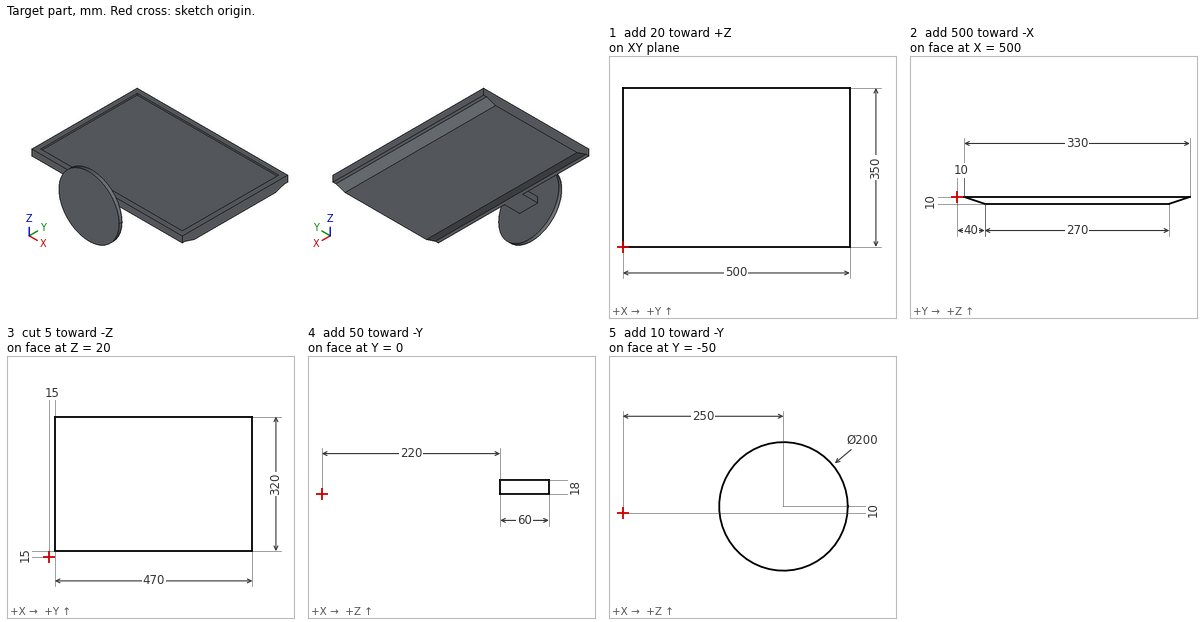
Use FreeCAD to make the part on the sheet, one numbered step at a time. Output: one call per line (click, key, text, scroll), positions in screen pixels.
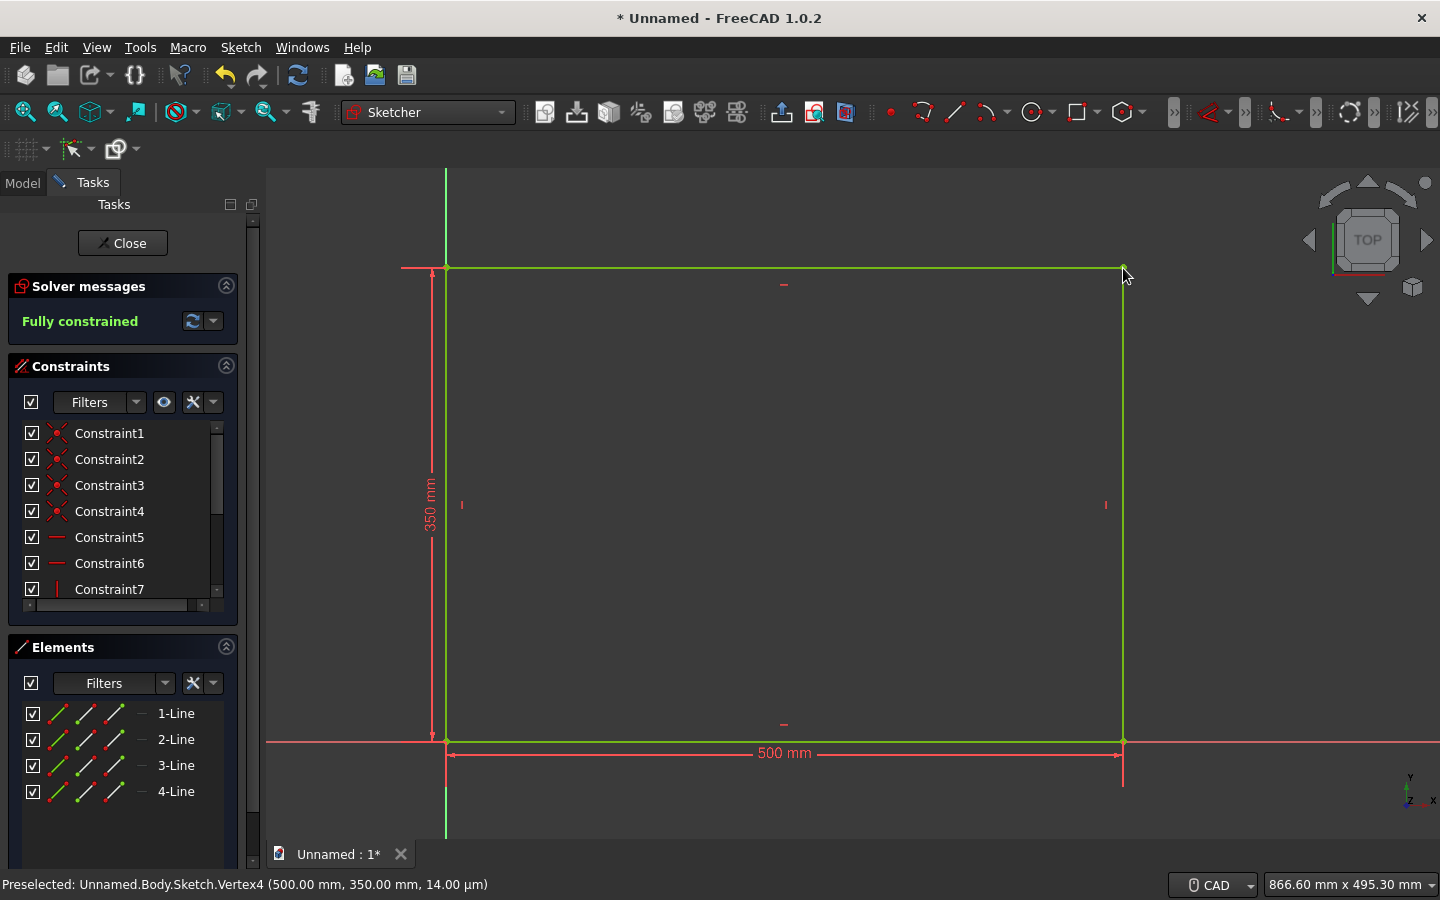
click(123, 243)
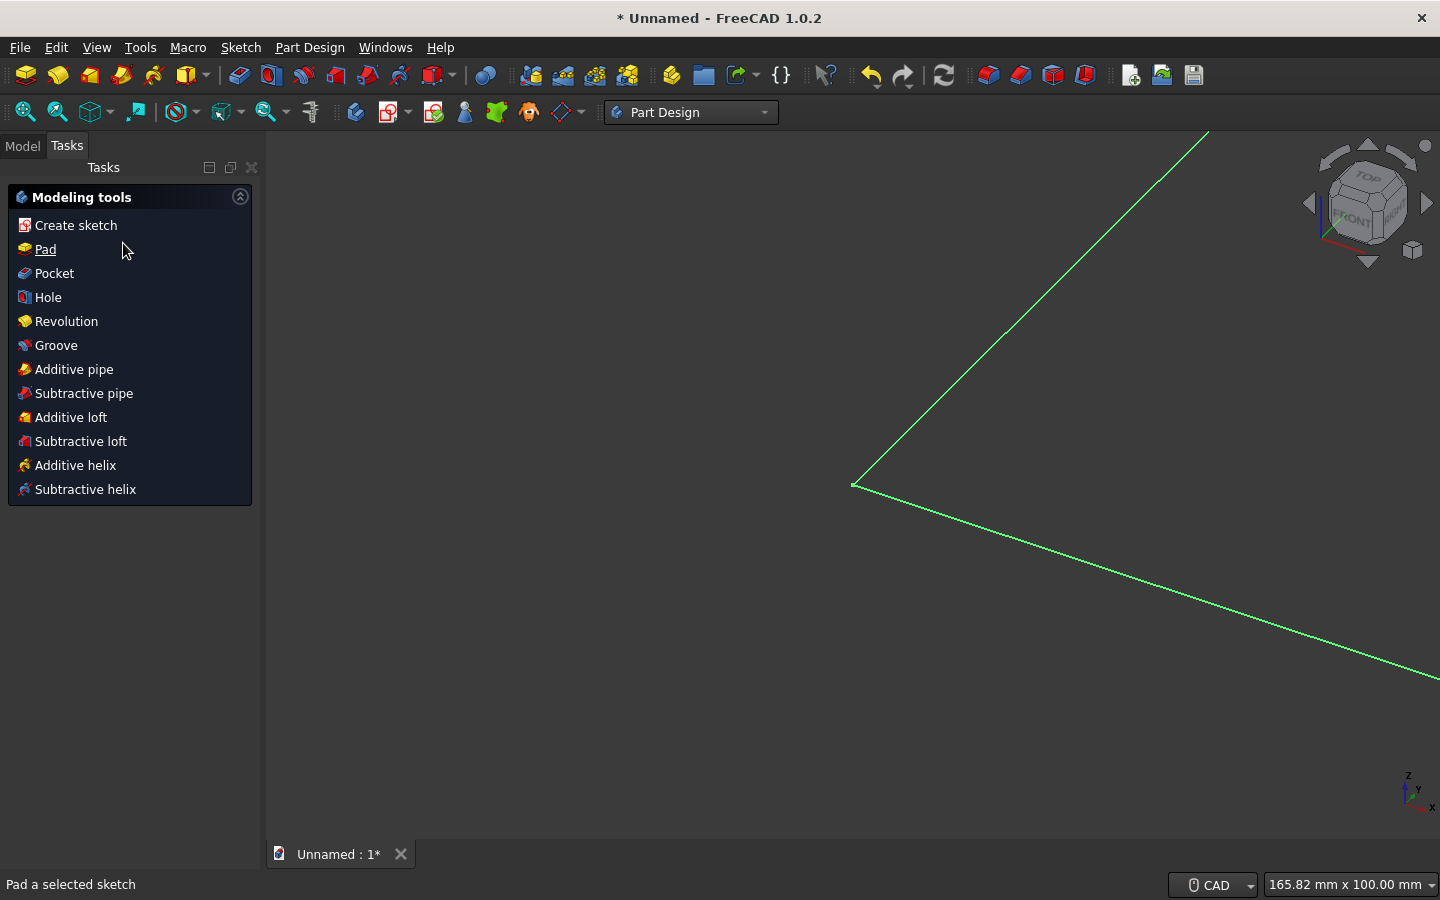
click(26, 76)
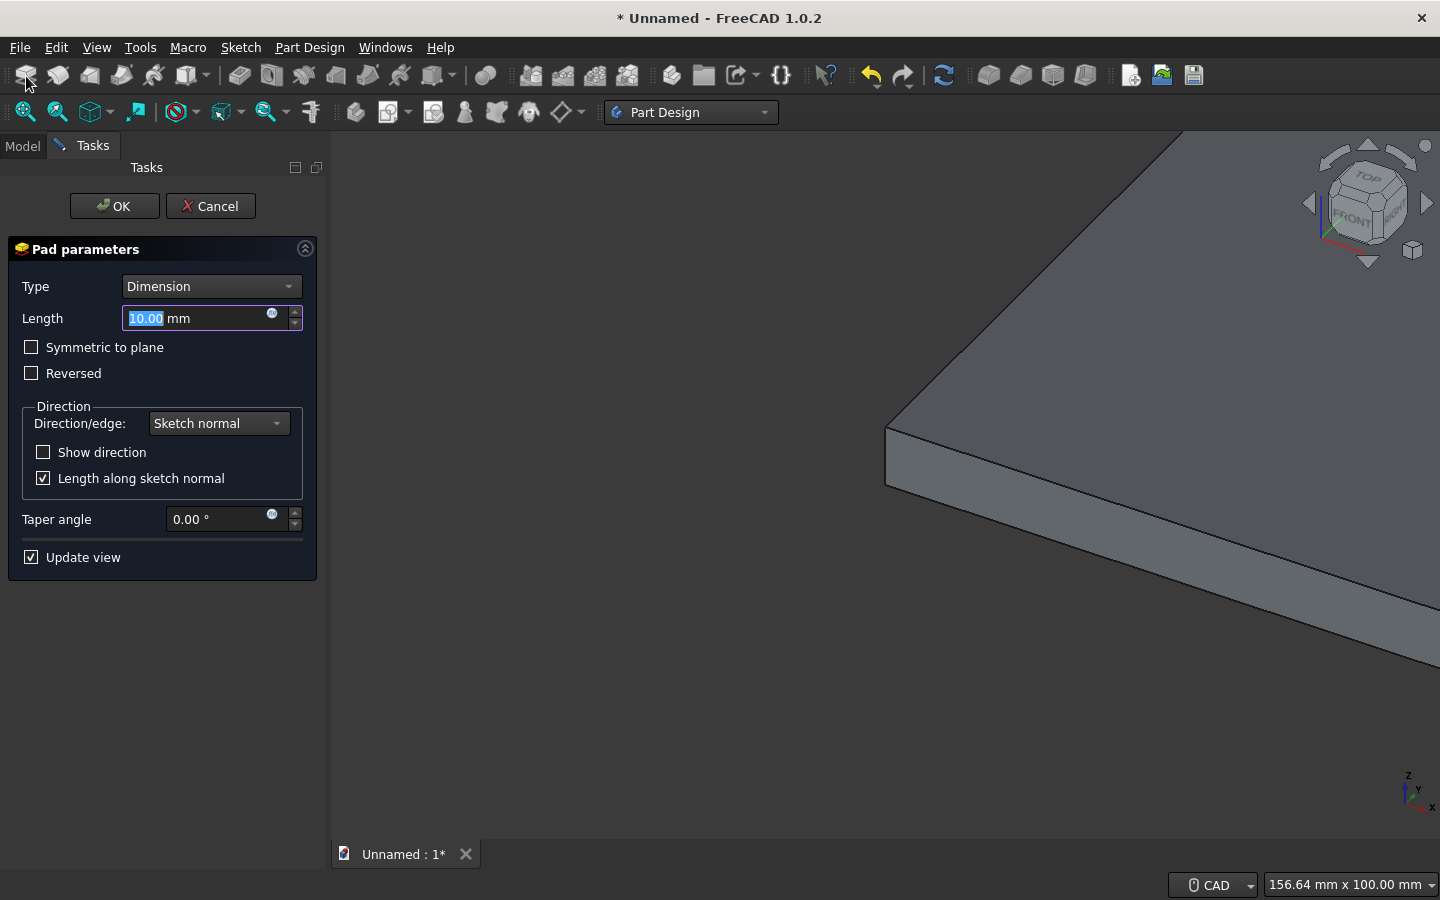
text(20)
key(Tab)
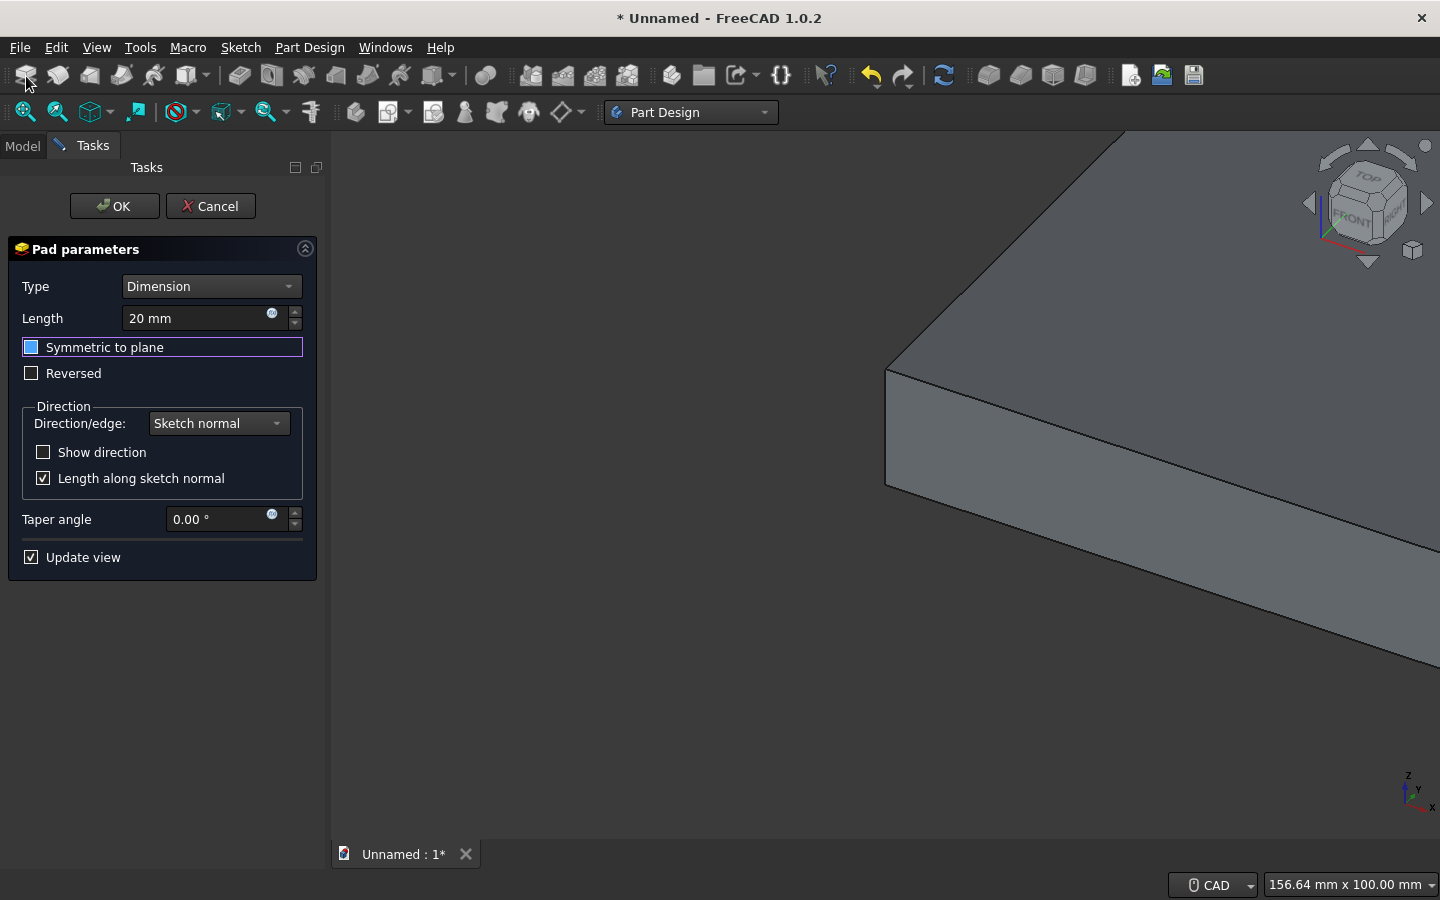
click(115, 206)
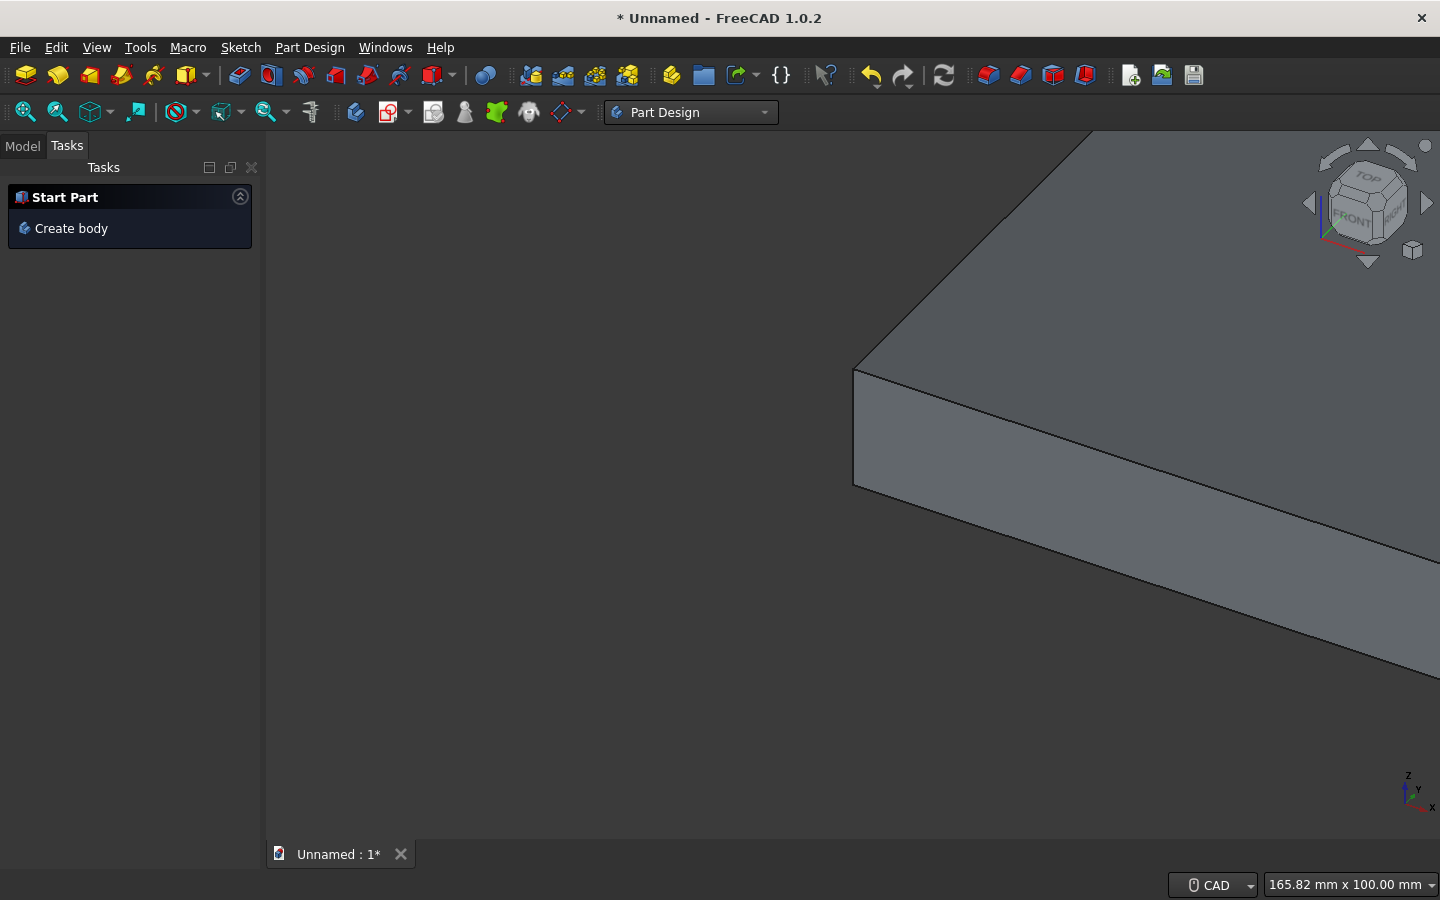
key(v)
key(f)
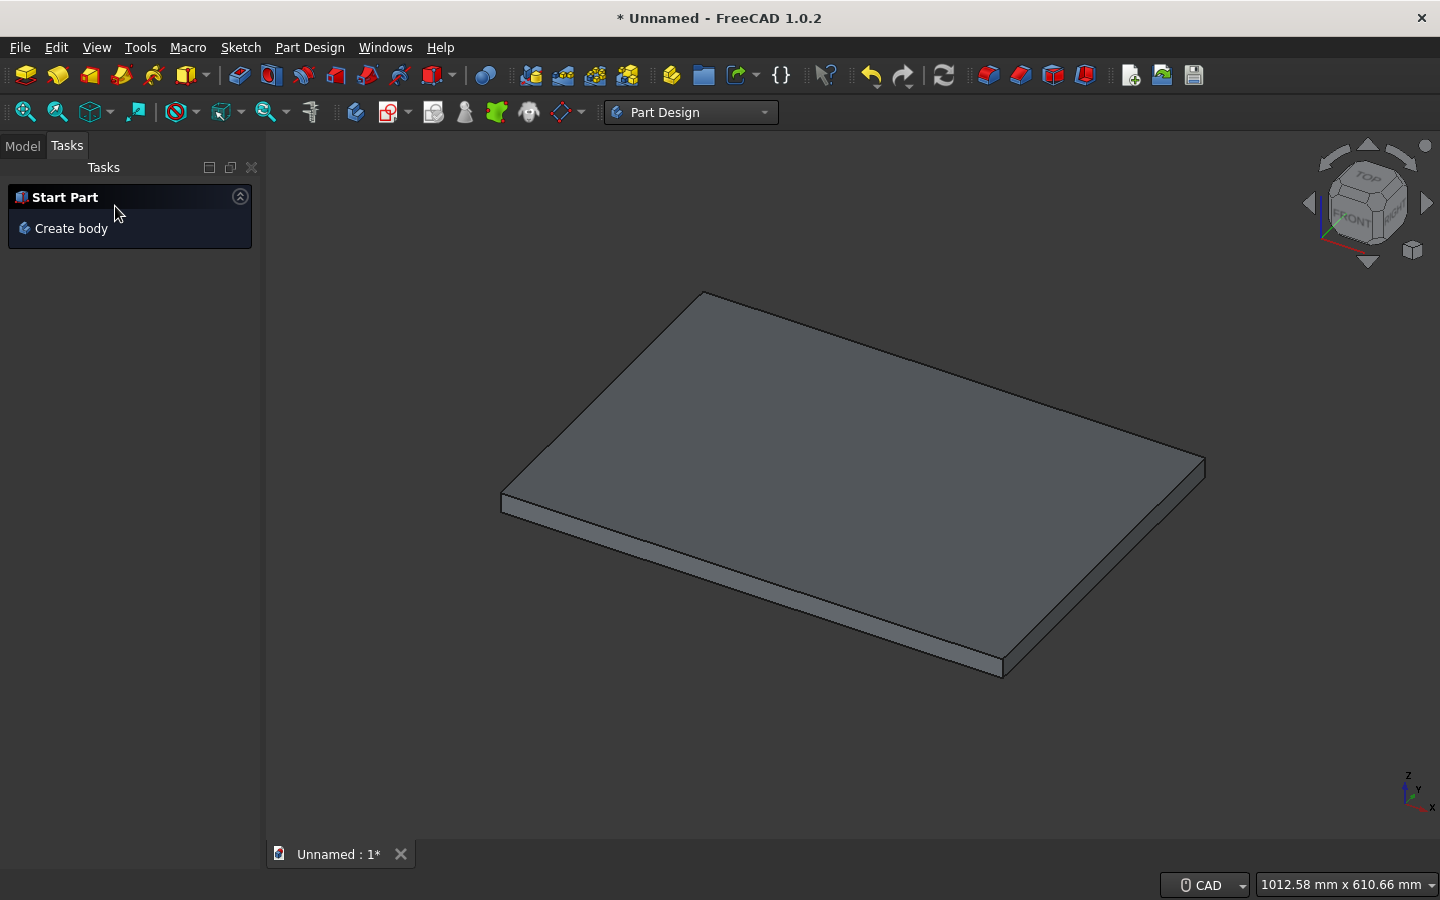
key(0)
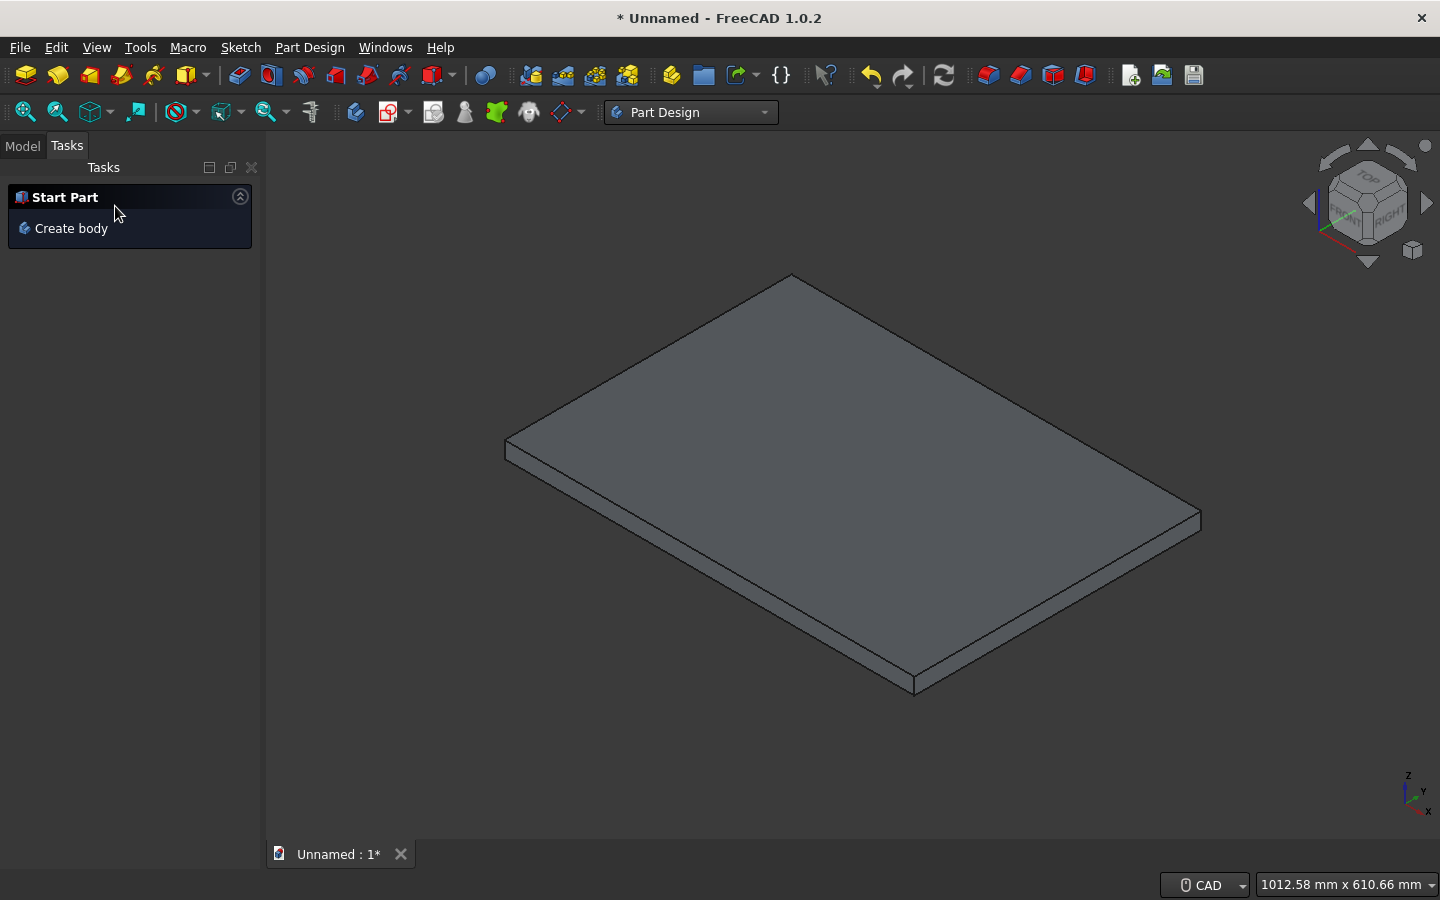
key(3)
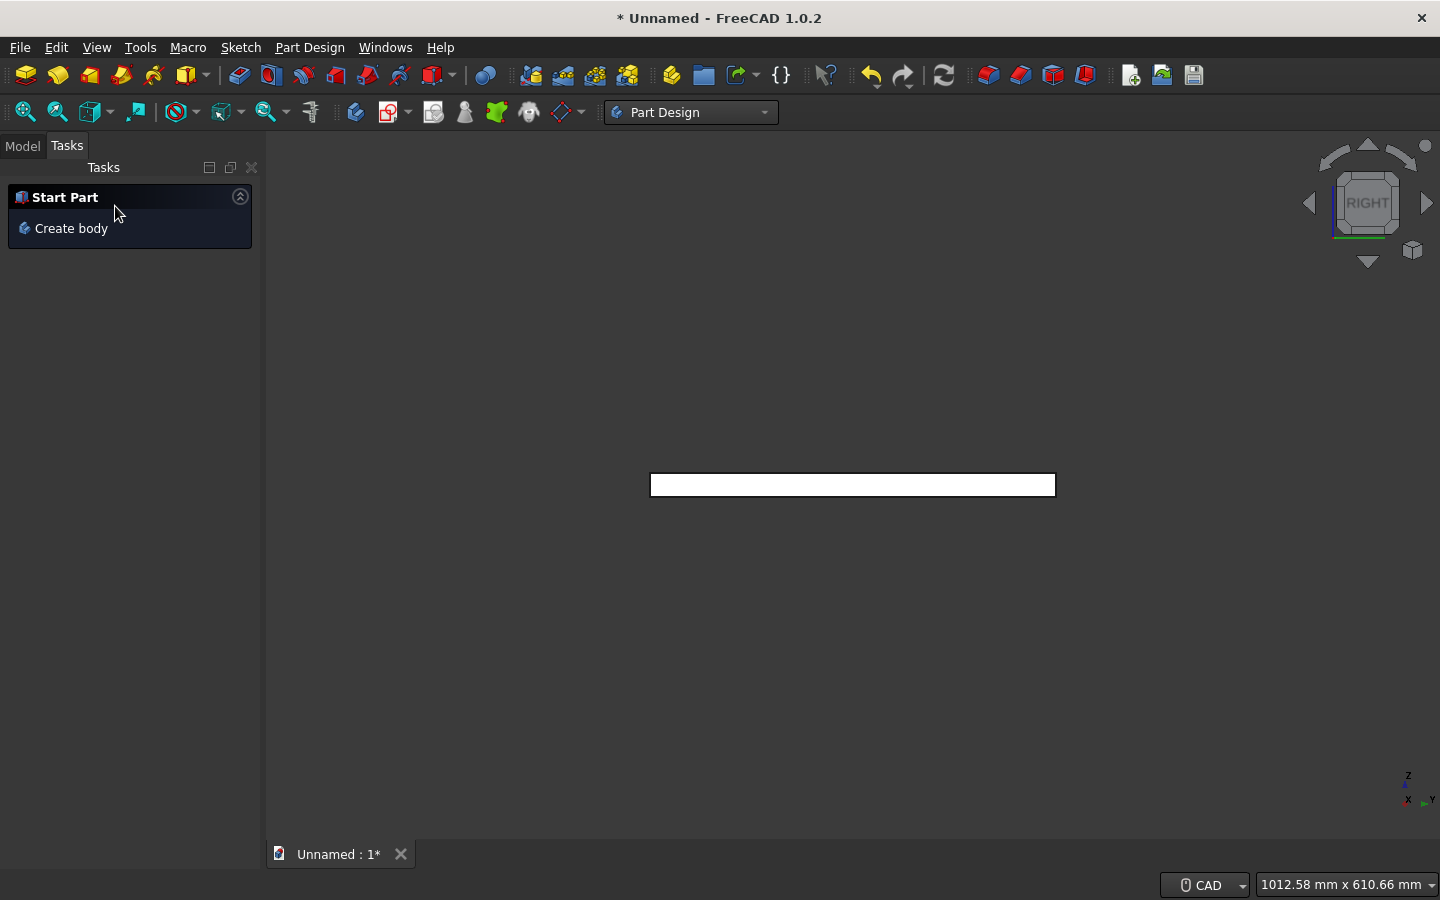
key(v)
key(f)